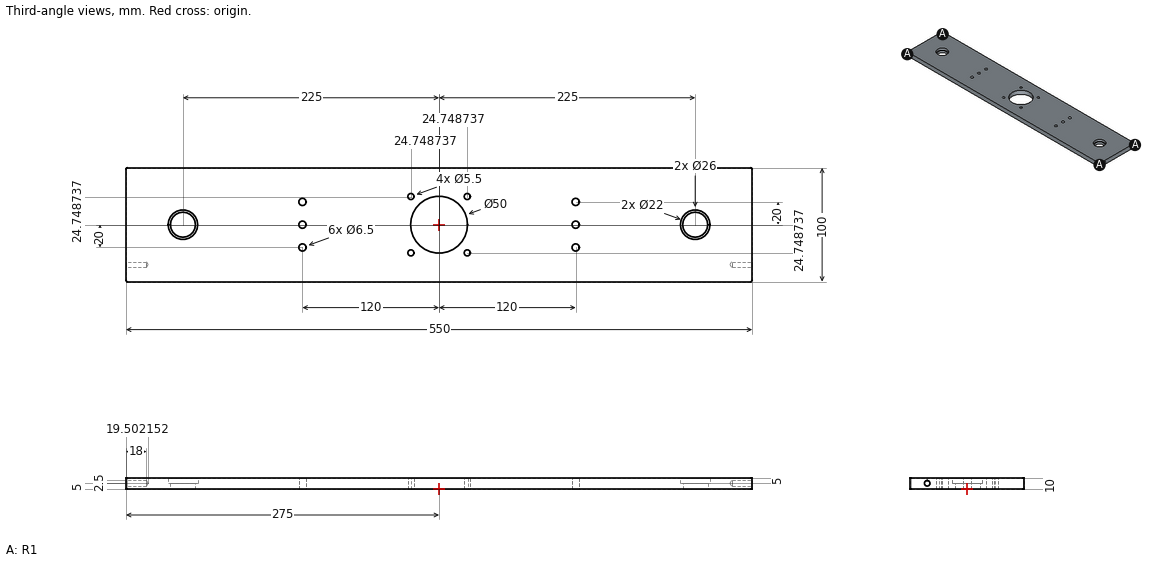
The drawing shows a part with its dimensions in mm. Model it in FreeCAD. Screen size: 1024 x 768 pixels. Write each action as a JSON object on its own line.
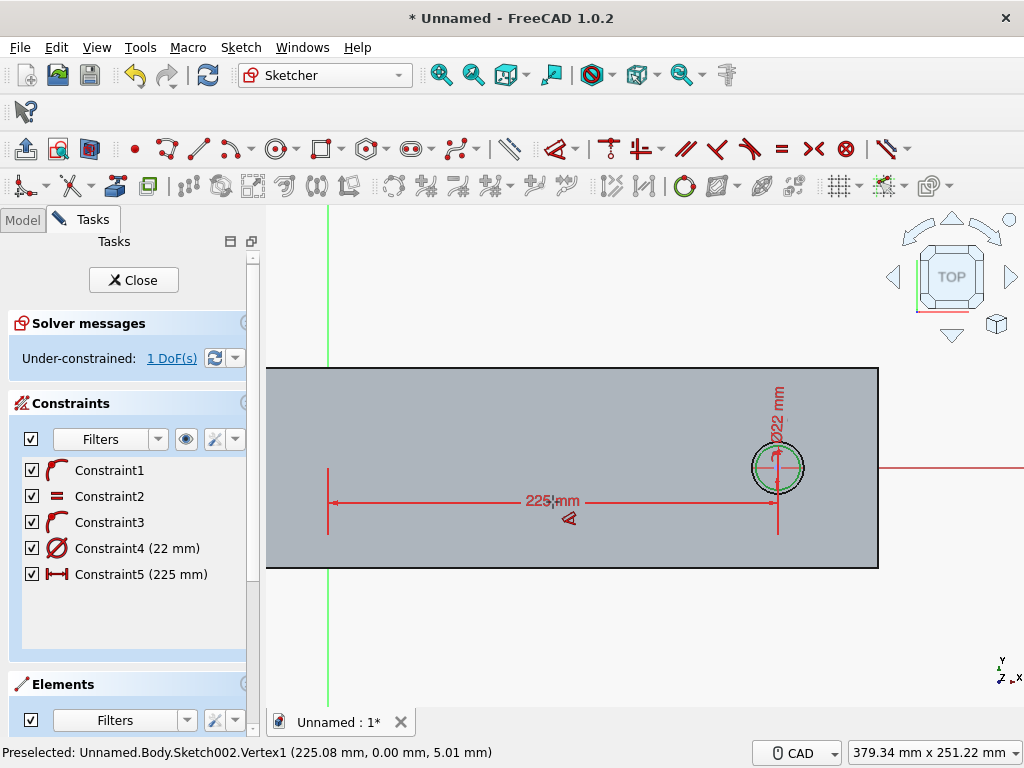
{"action": "scroll", "coordinate": [779, 446], "scroll_direction": "down", "scroll_amount": 4}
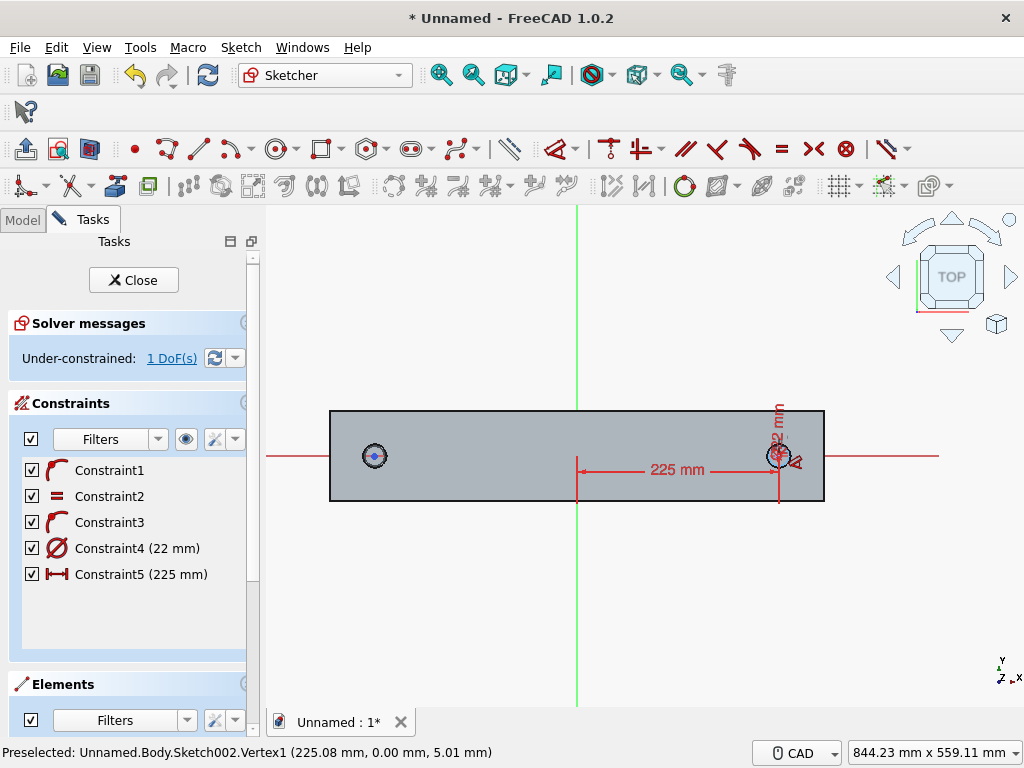
{"action": "left_click", "coordinate": [375, 456]}
{"action": "left_click", "coordinate": [476, 490]}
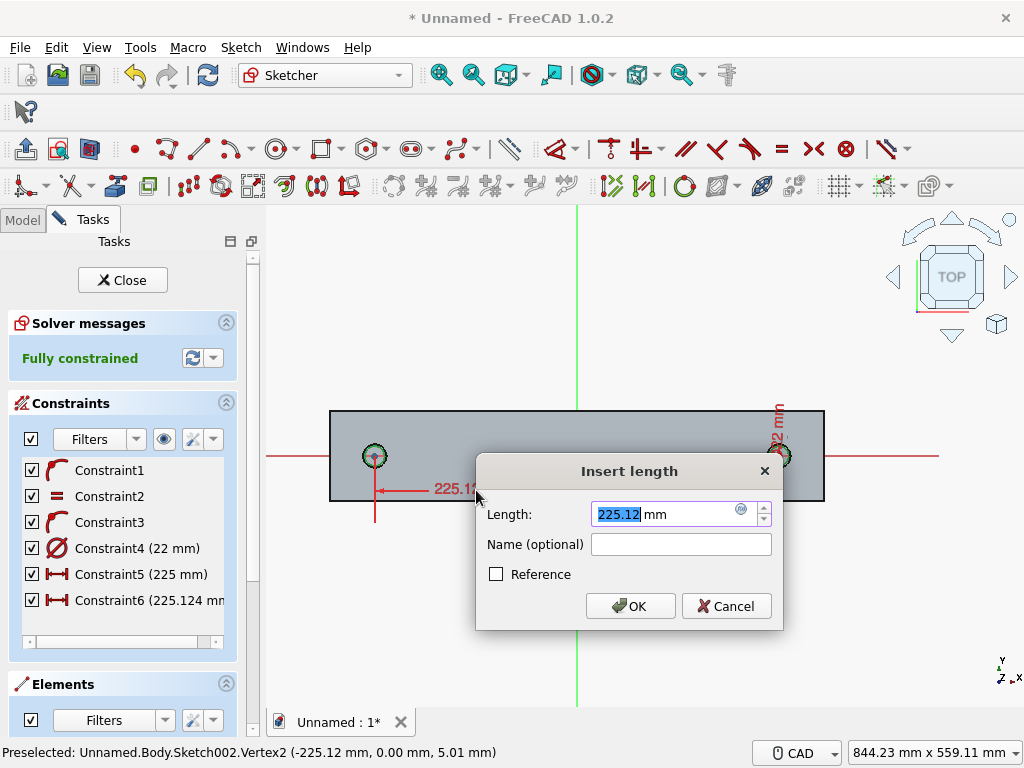
{"action": "type", "text": "225"}
{"action": "key", "text": "Return"}
{"action": "key", "text": "Escape"}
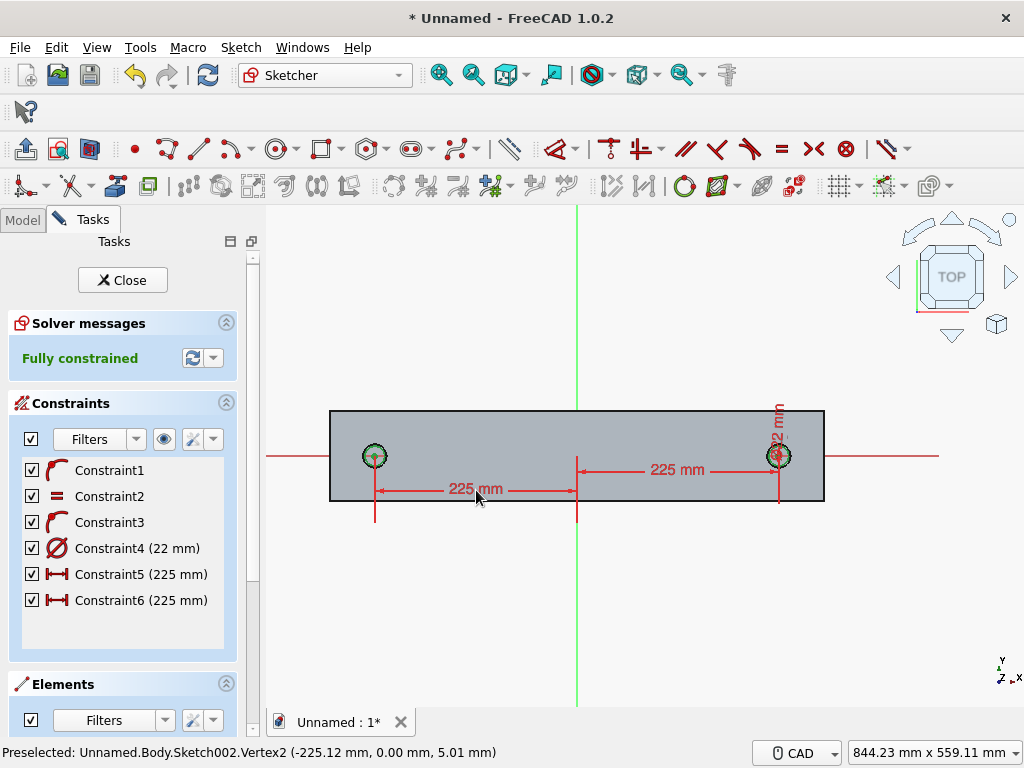
{"action": "left_click", "coordinate": [123, 280]}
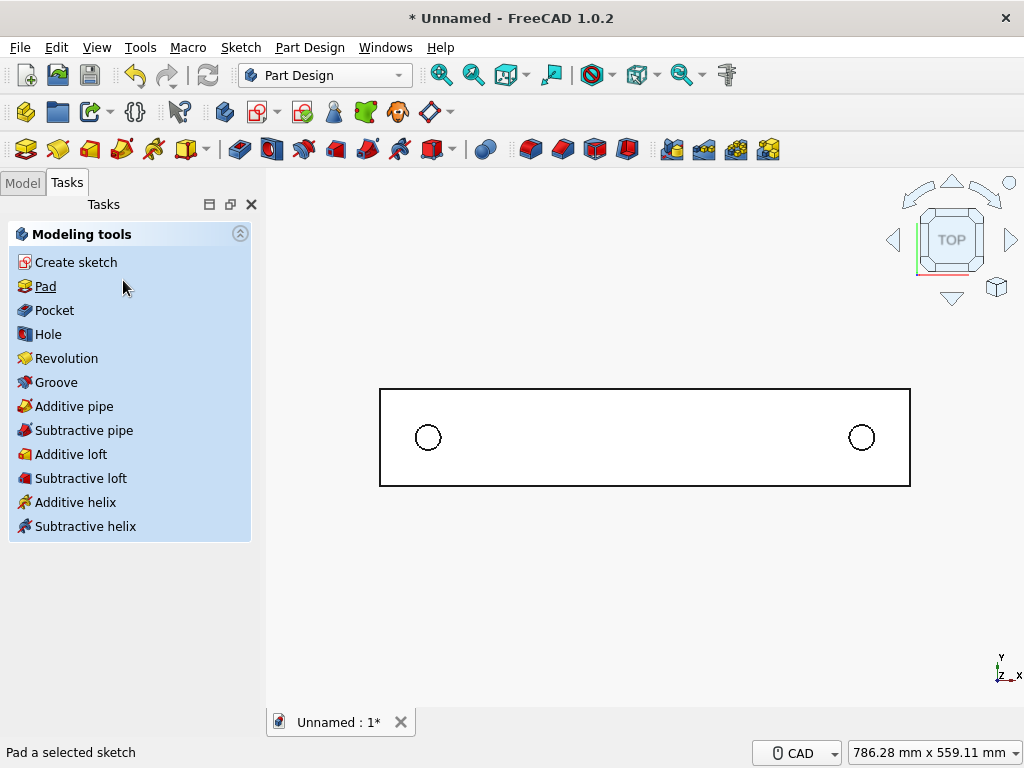
{"action": "left_click", "coordinate": [240, 150]}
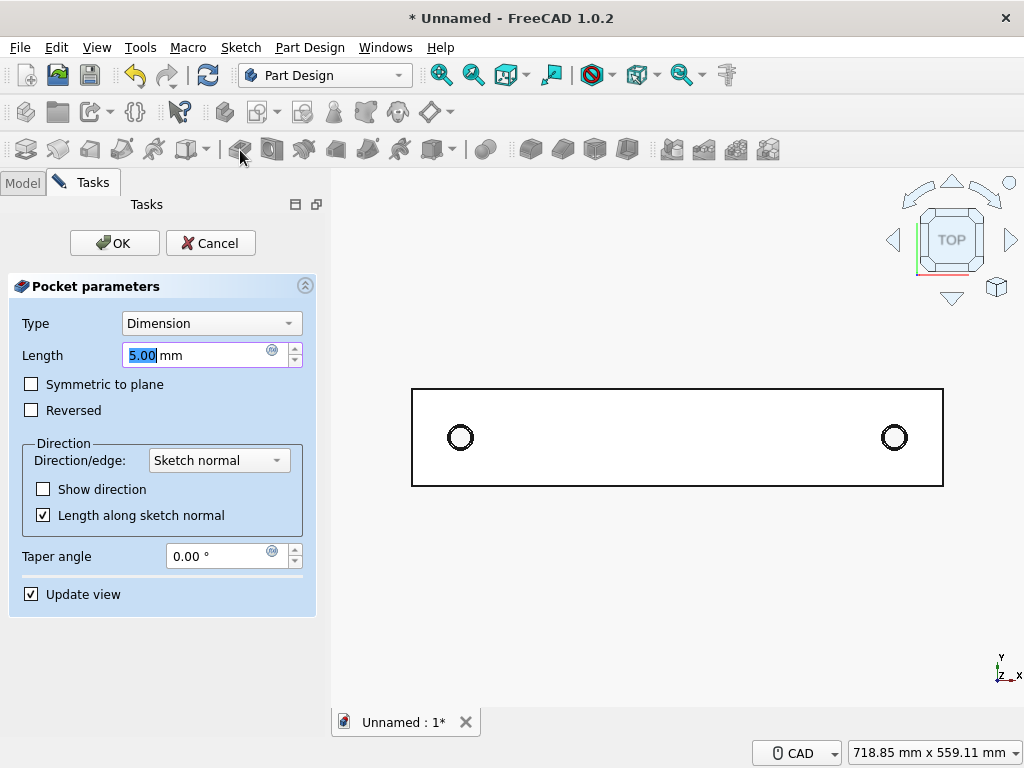
{"action": "left_click", "coordinate": [212, 324]}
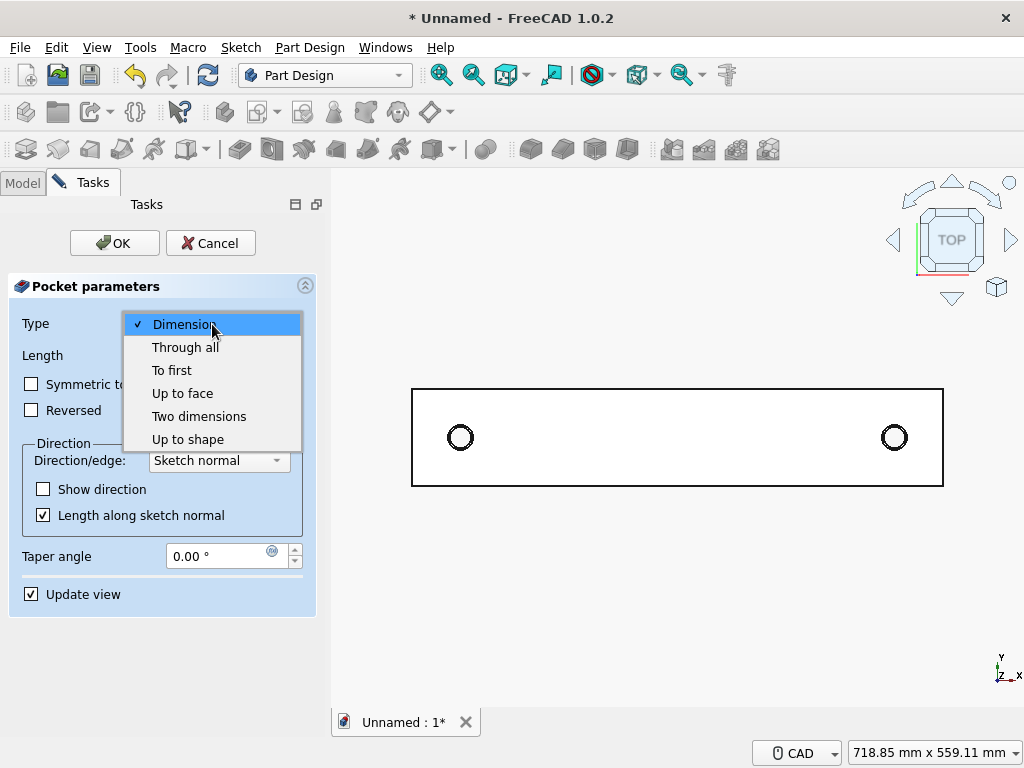
{"action": "left_click", "coordinate": [212, 348]}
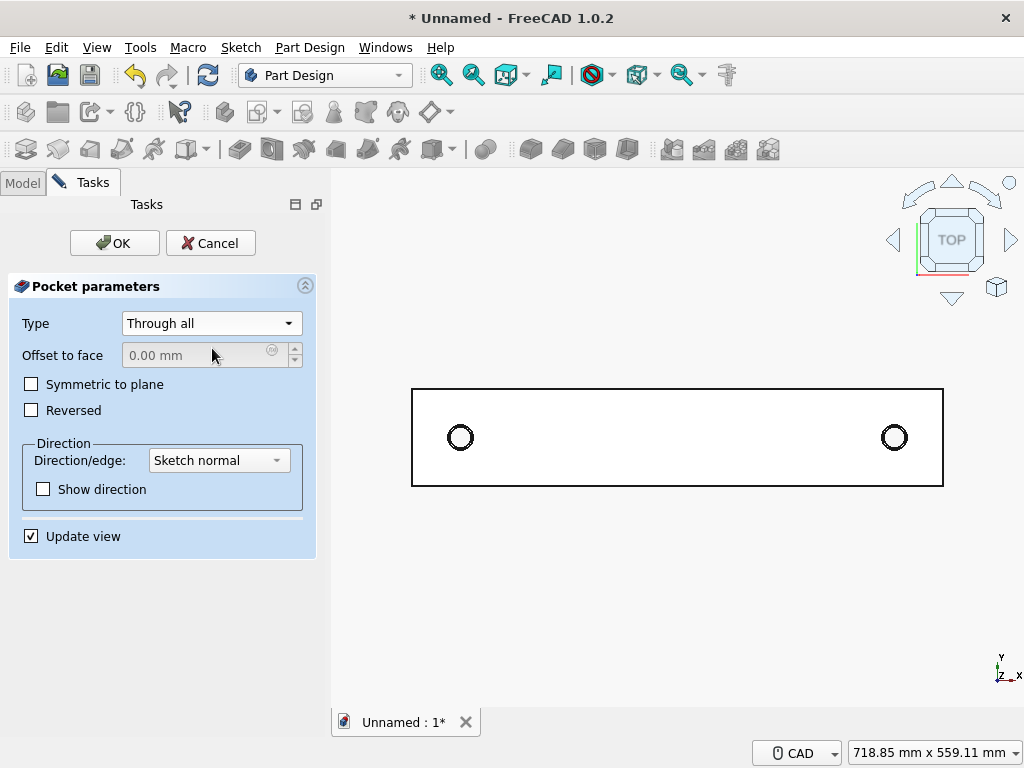
{"action": "left_click", "coordinate": [115, 243]}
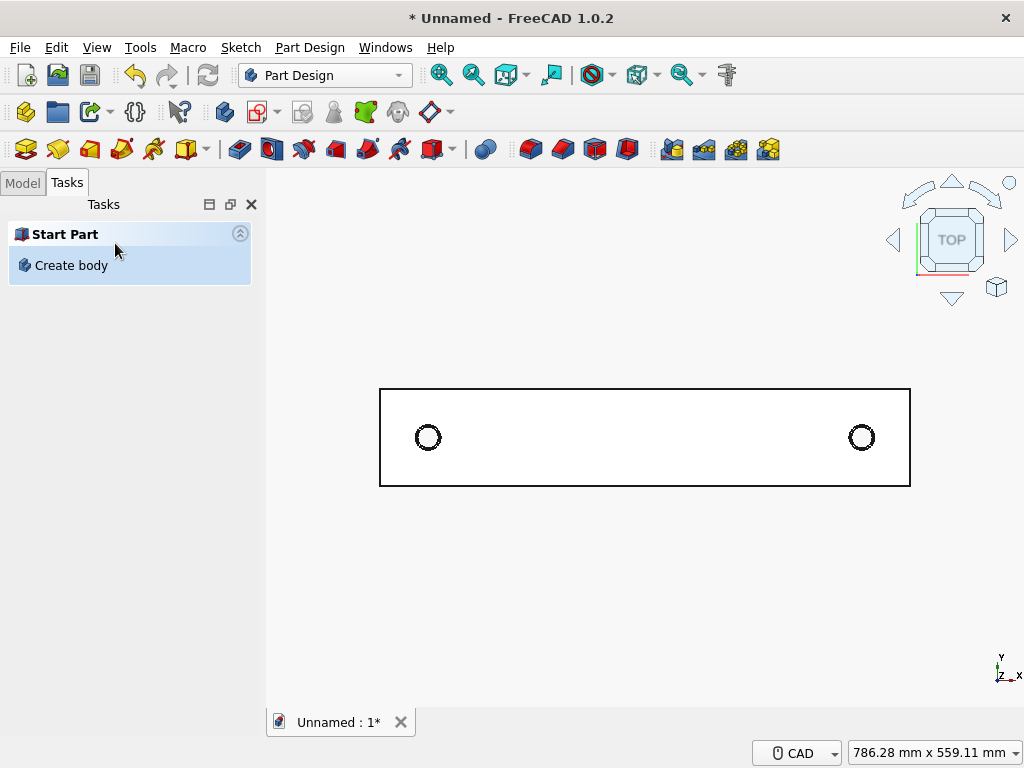
{"action": "left_click", "coordinate": [796, 437]}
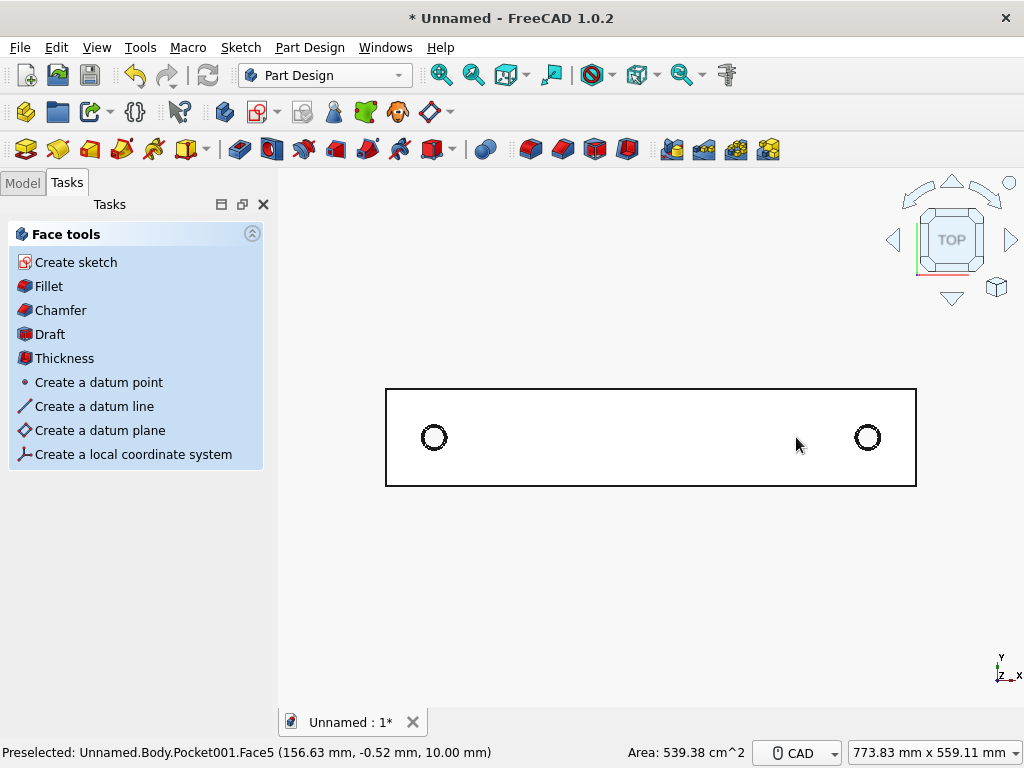
{"action": "left_click", "coordinate": [258, 112]}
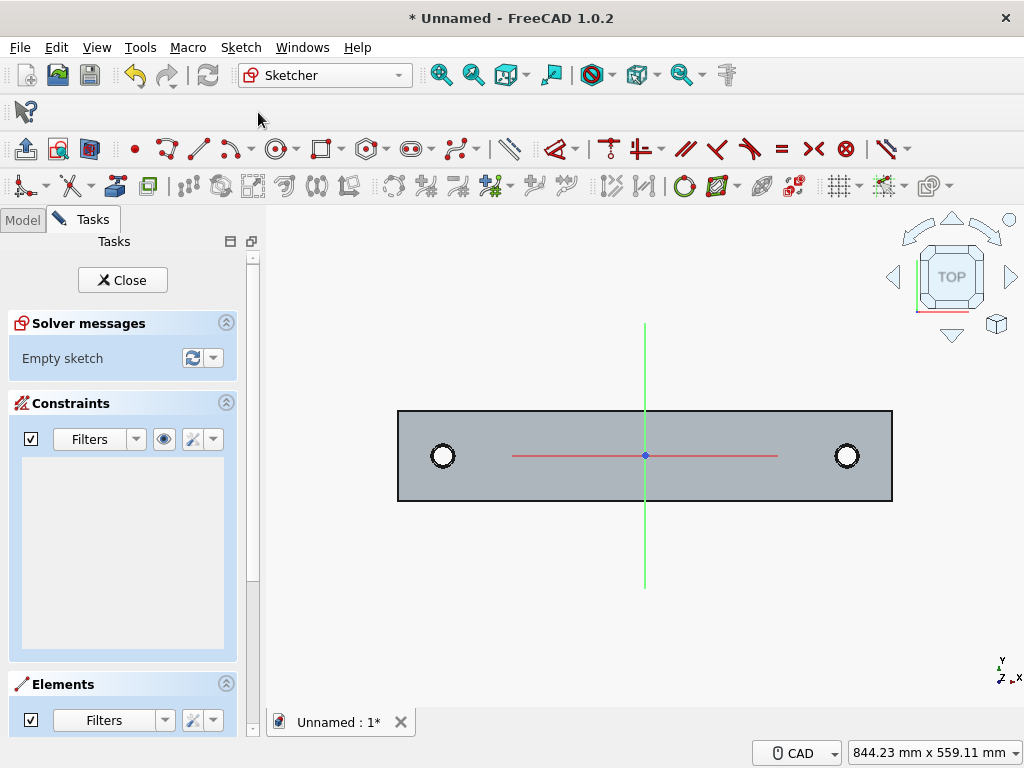
{"action": "scroll", "coordinate": [656, 456], "scroll_direction": "up", "scroll_amount": 10}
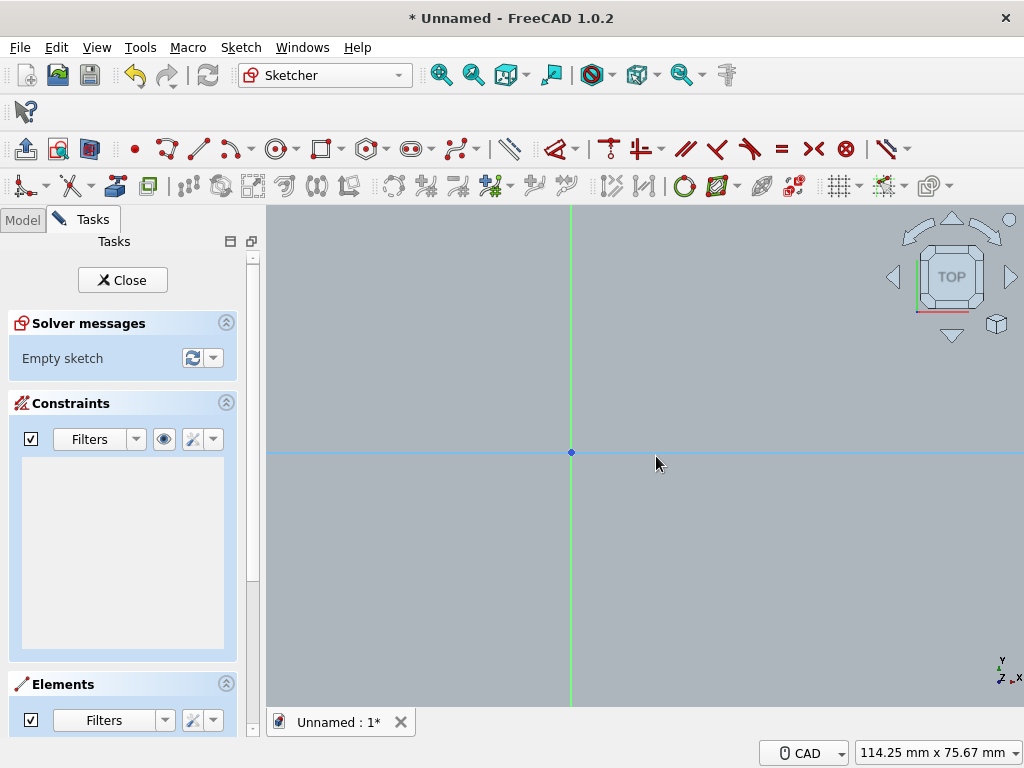
{"action": "key", "text": "g c"}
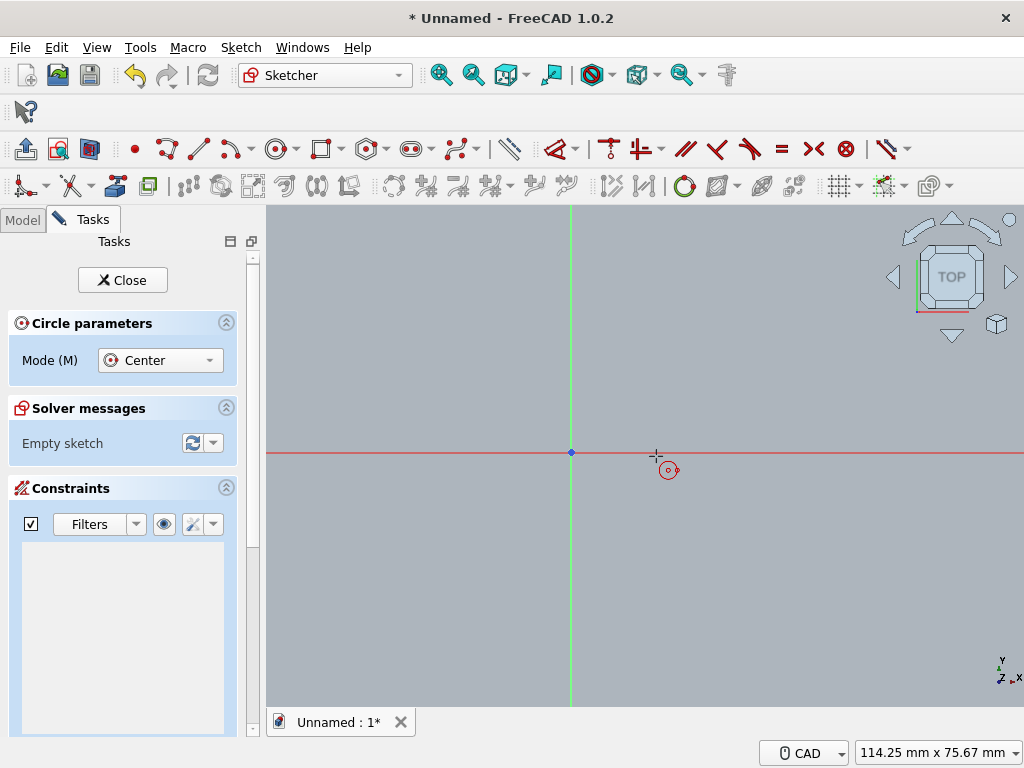
{"action": "left_click", "coordinate": [571, 453]}
{"action": "left_click", "coordinate": [689, 336]}
{"action": "key", "text": "Escape"}